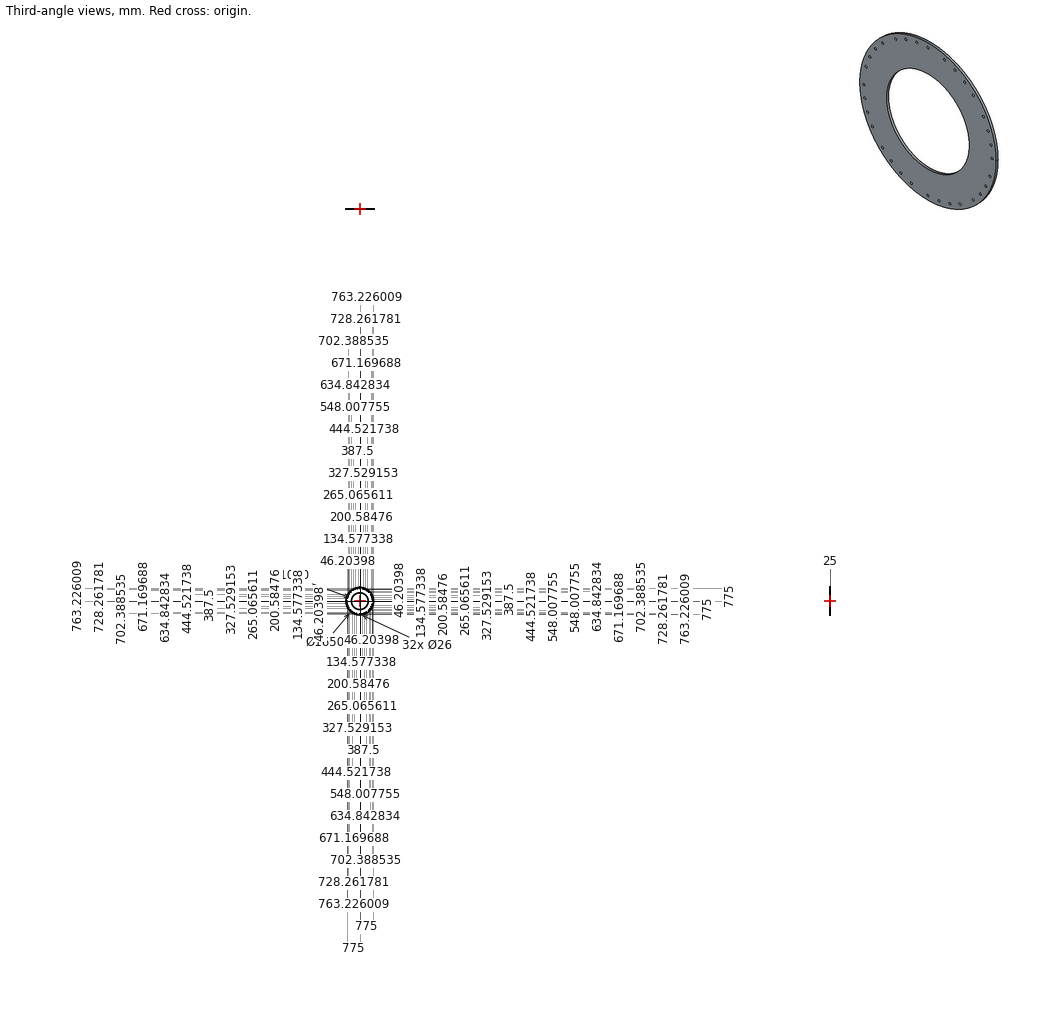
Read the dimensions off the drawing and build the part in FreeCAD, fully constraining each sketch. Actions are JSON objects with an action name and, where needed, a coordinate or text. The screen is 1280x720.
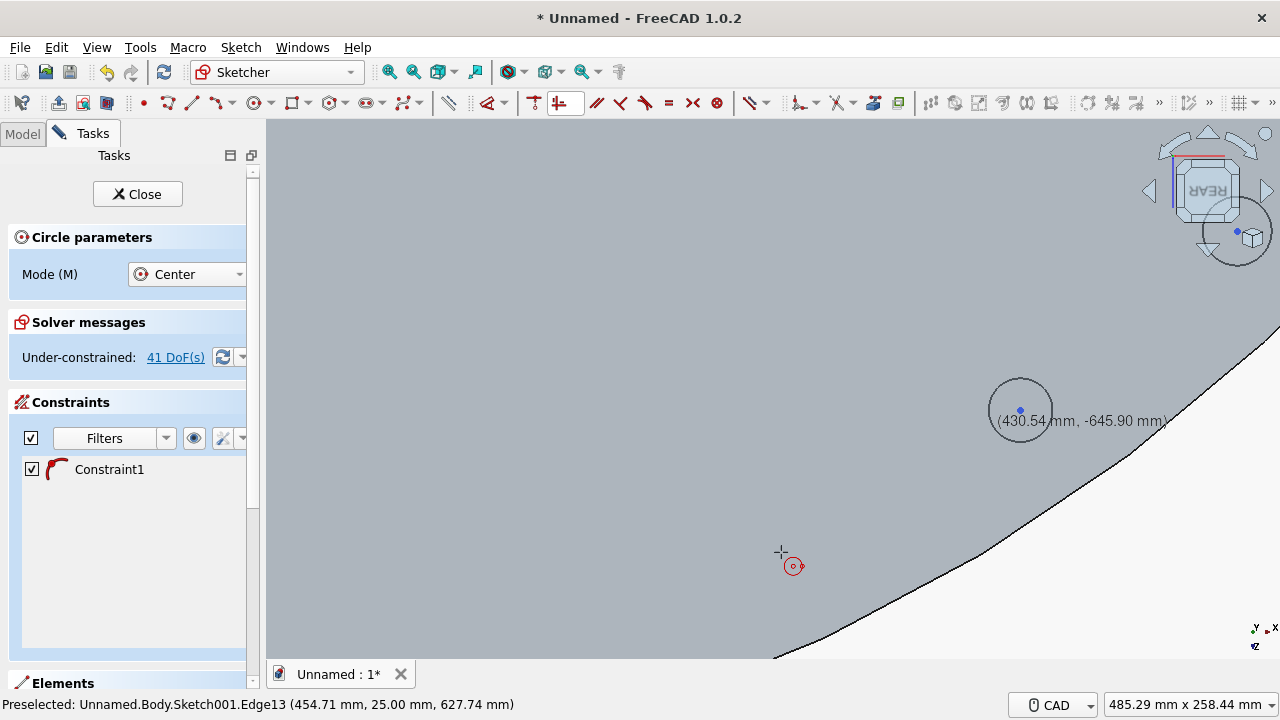
{"action": "scroll", "coordinate": [781, 553], "scroll_direction": "down", "scroll_amount": 11}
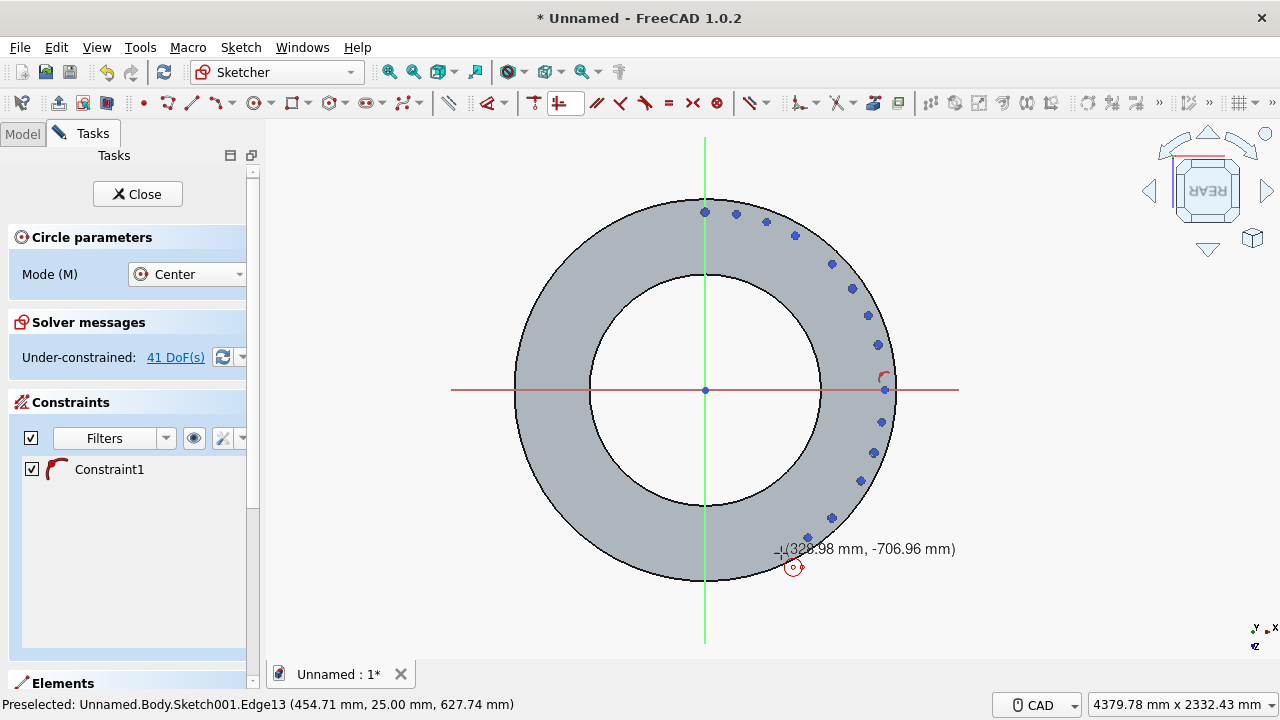
{"action": "left_click", "coordinate": [781, 553]}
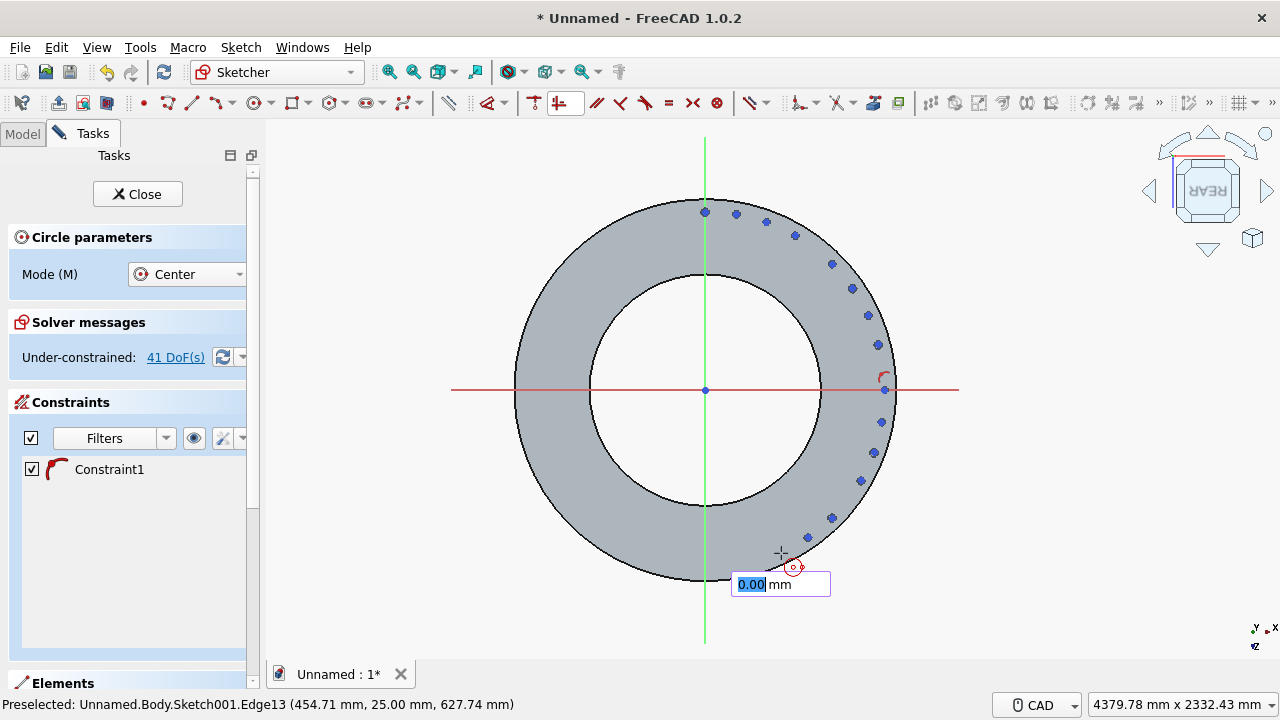
{"action": "scroll", "coordinate": [783, 551], "scroll_direction": "up", "scroll_amount": 9}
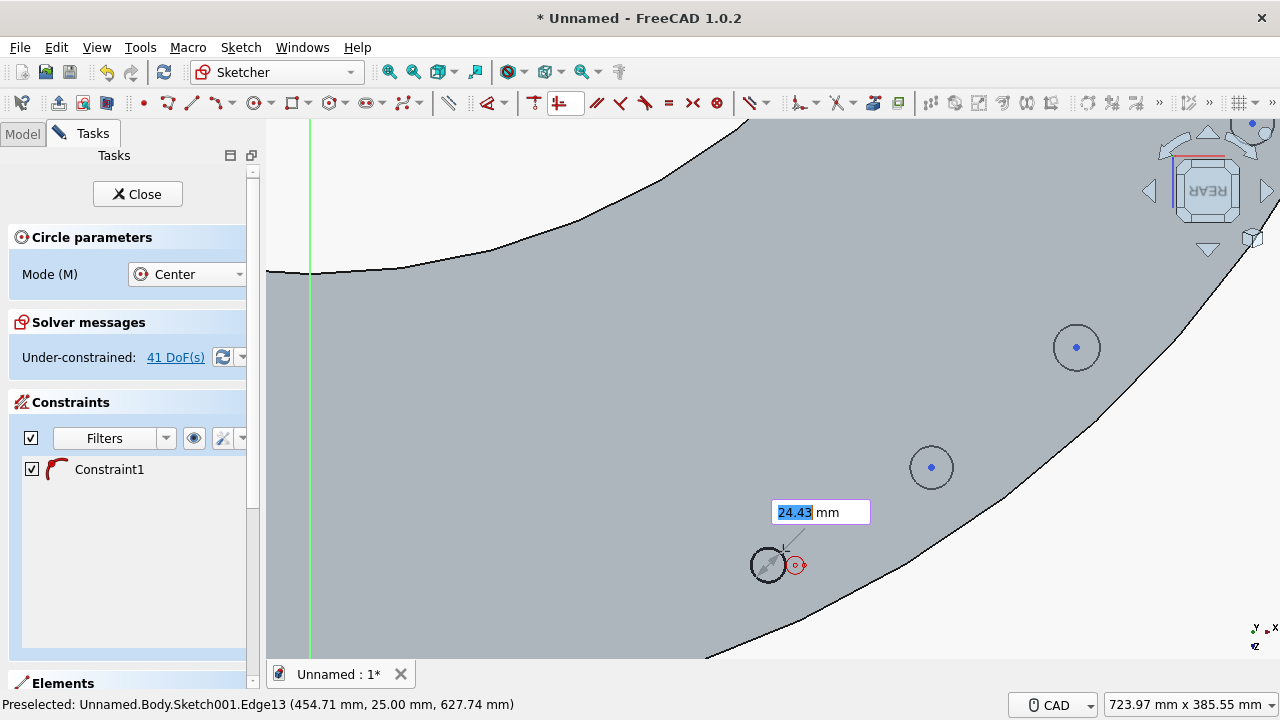
{"action": "left_click", "coordinate": [782, 545]}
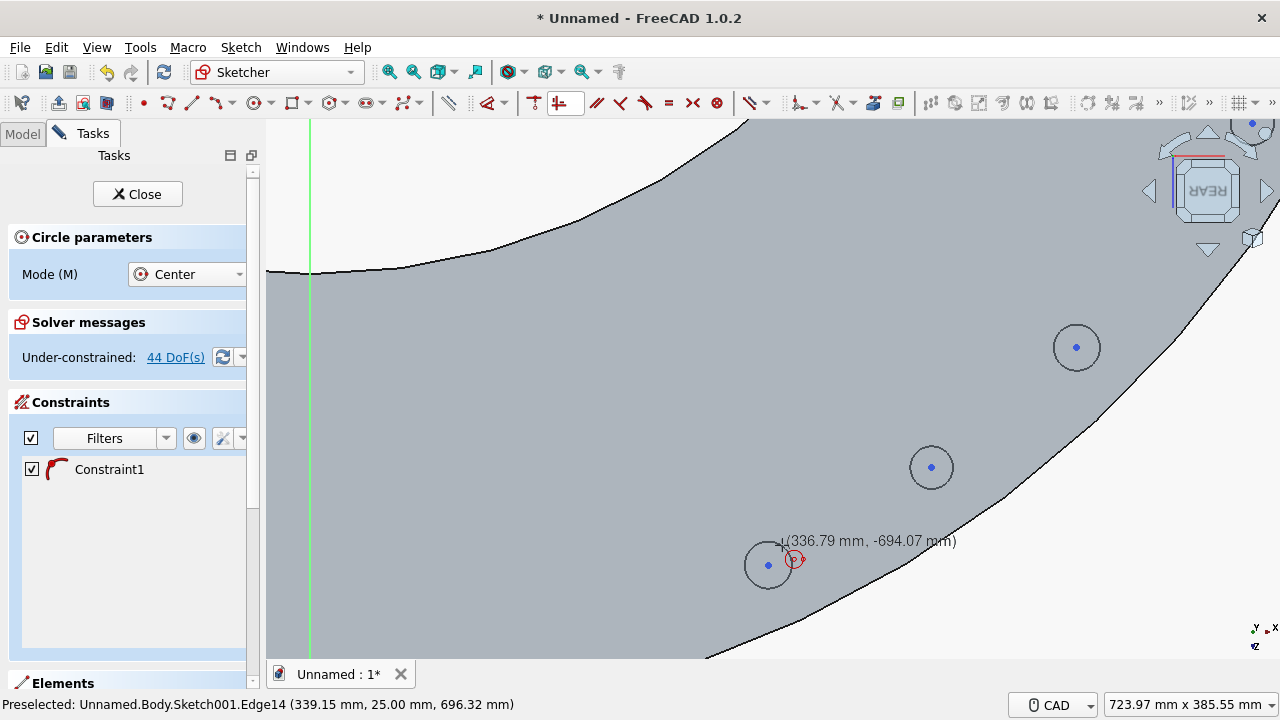
{"action": "scroll", "coordinate": [591, 622], "scroll_direction": "up", "scroll_amount": 2}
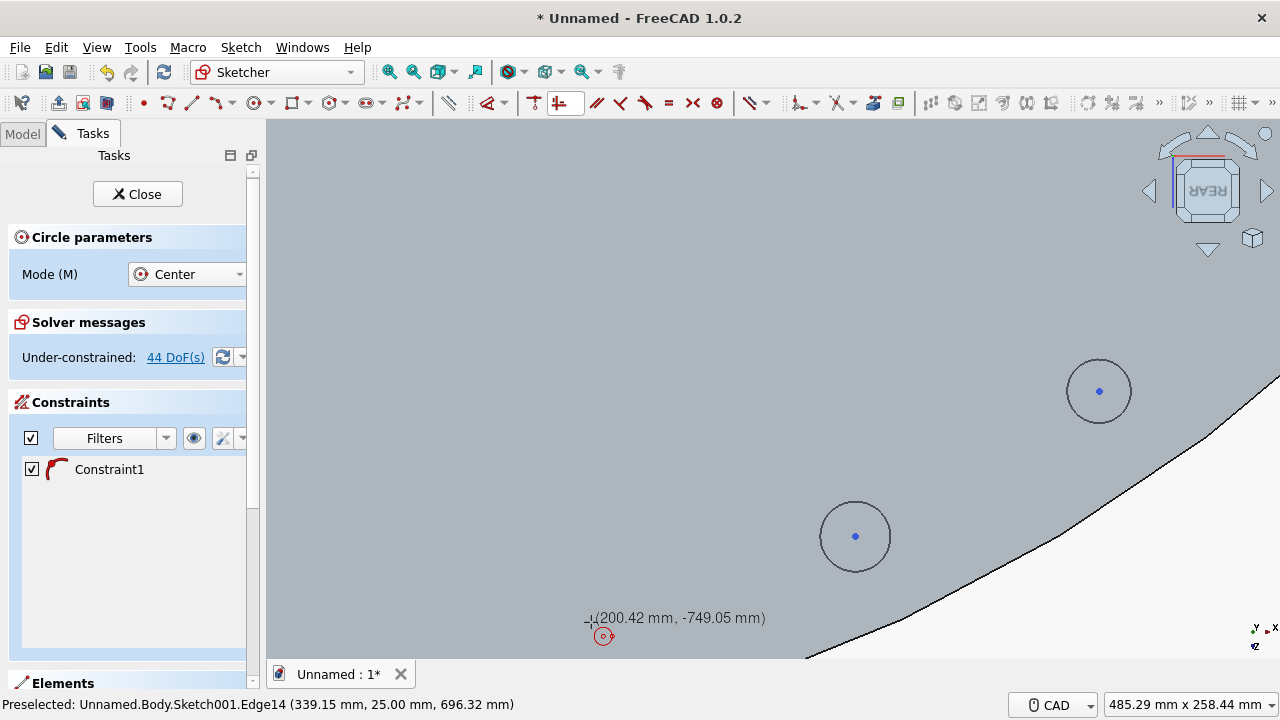
{"action": "scroll", "coordinate": [771, 555], "scroll_direction": "down", "scroll_amount": 11}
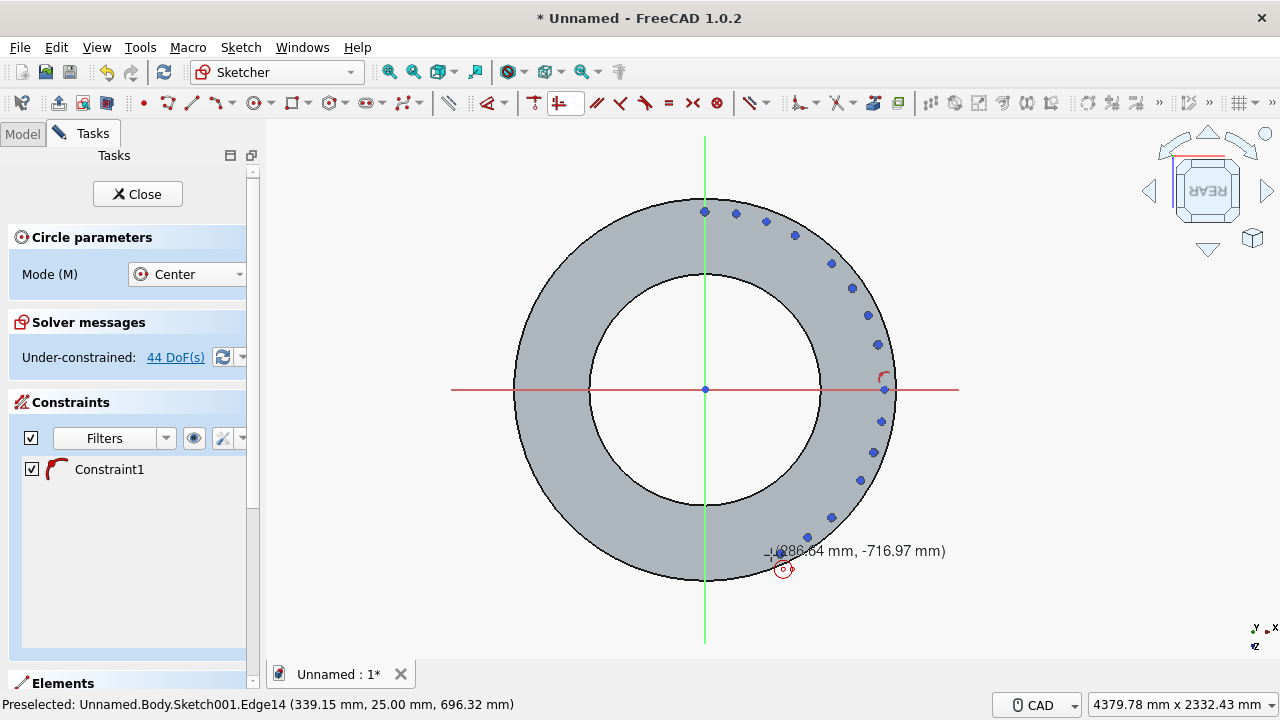
{"action": "left_click", "coordinate": [752, 563]}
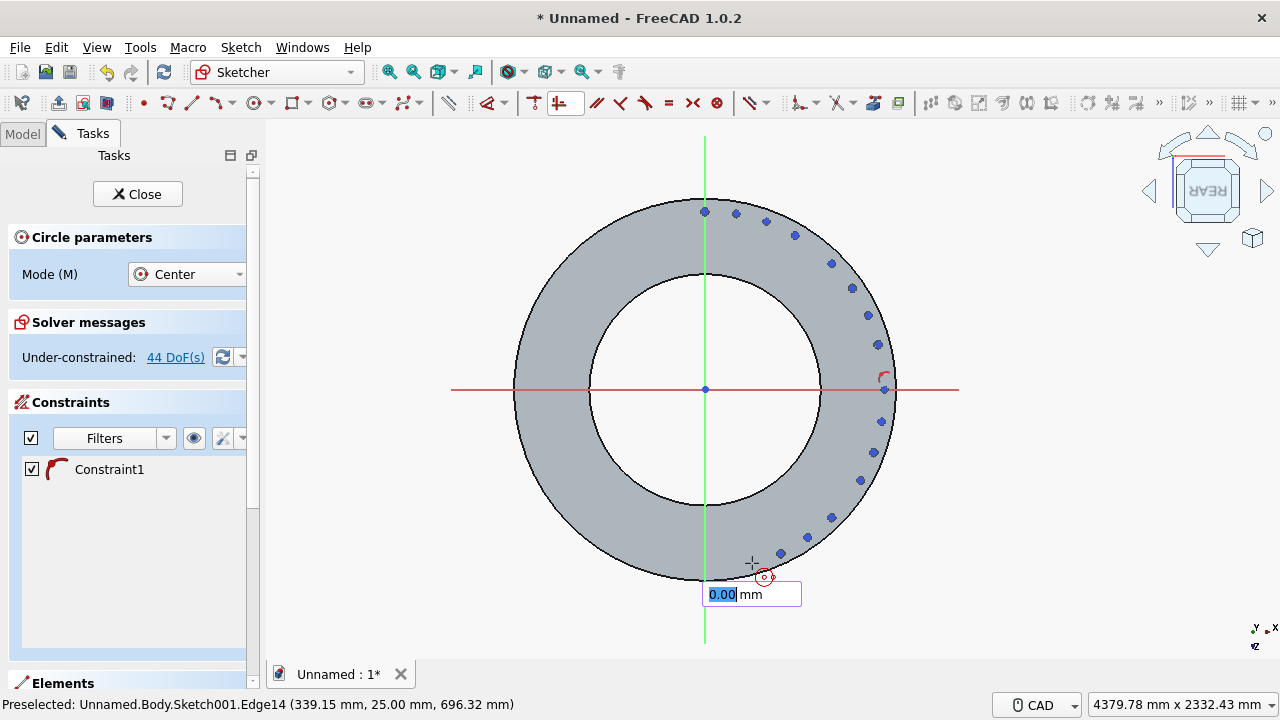
{"action": "scroll", "coordinate": [754, 561], "scroll_direction": "up", "scroll_amount": 9}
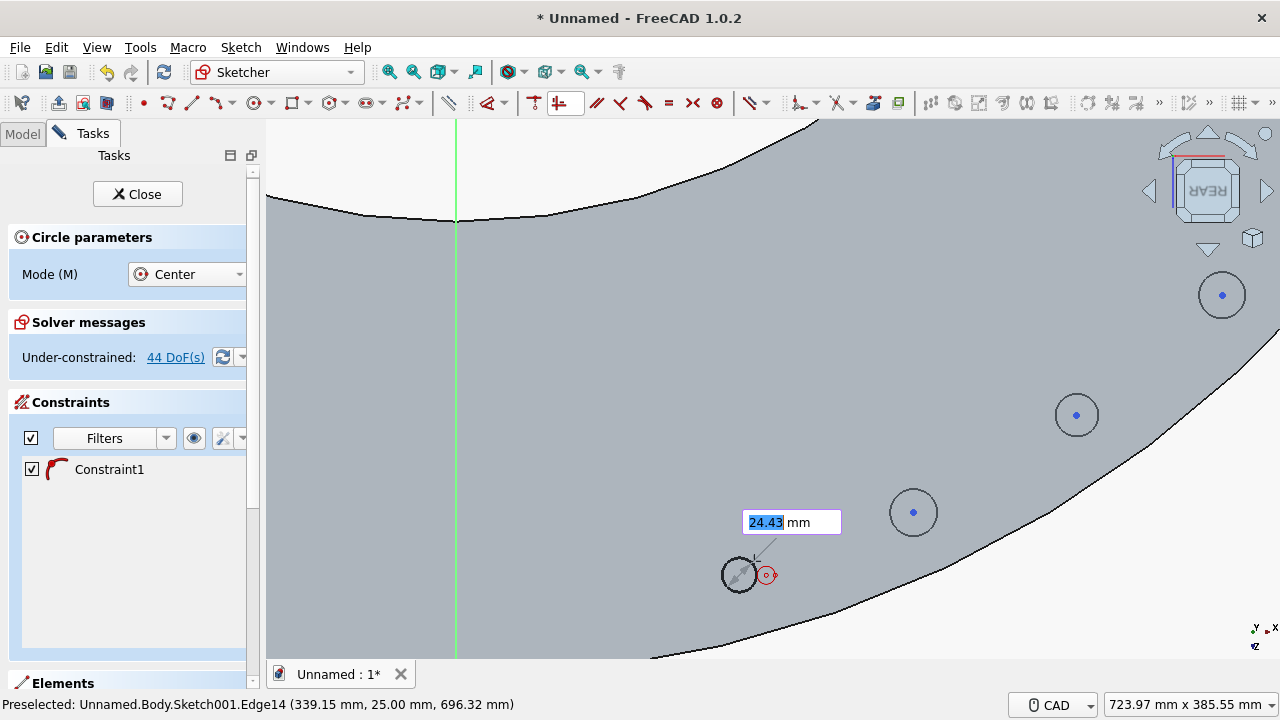
{"action": "left_click", "coordinate": [749, 557]}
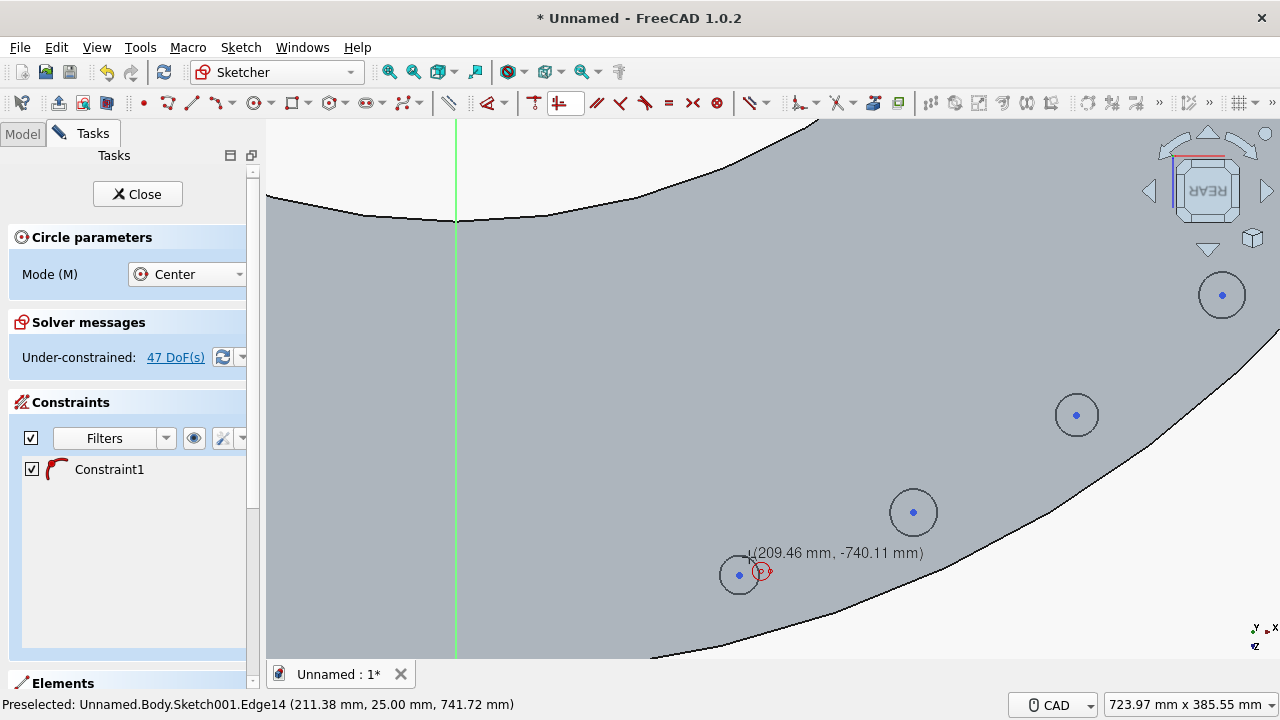
{"action": "scroll", "coordinate": [456, 607], "scroll_direction": "up", "scroll_amount": 2}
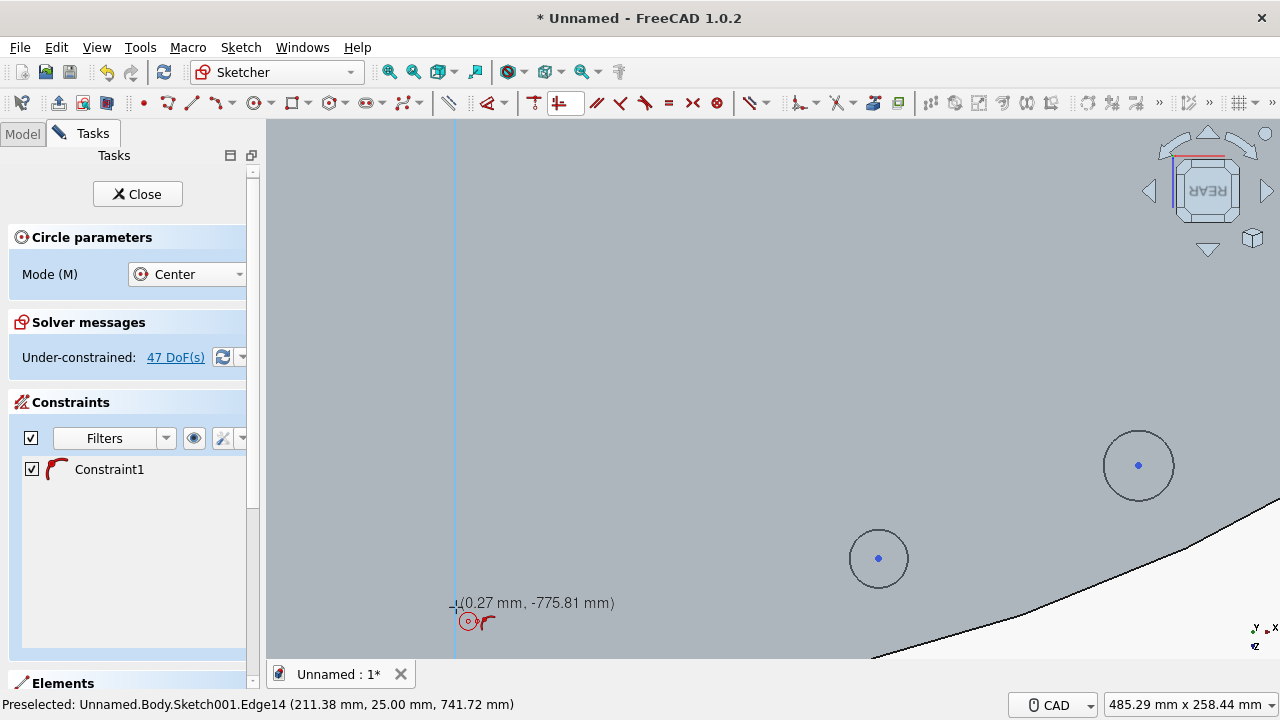
{"action": "scroll", "coordinate": [736, 564], "scroll_direction": "down", "scroll_amount": 11}